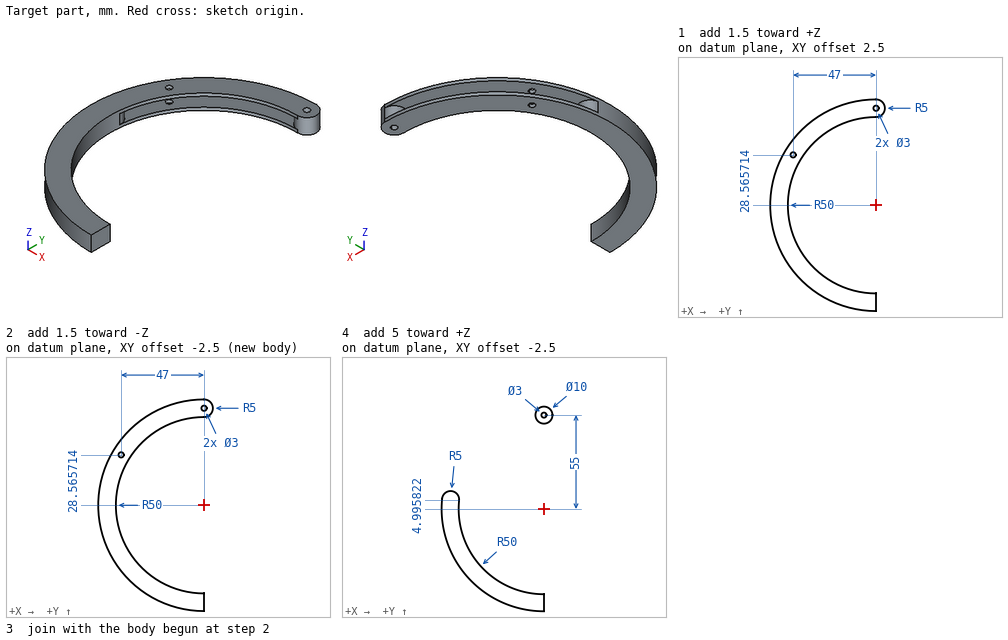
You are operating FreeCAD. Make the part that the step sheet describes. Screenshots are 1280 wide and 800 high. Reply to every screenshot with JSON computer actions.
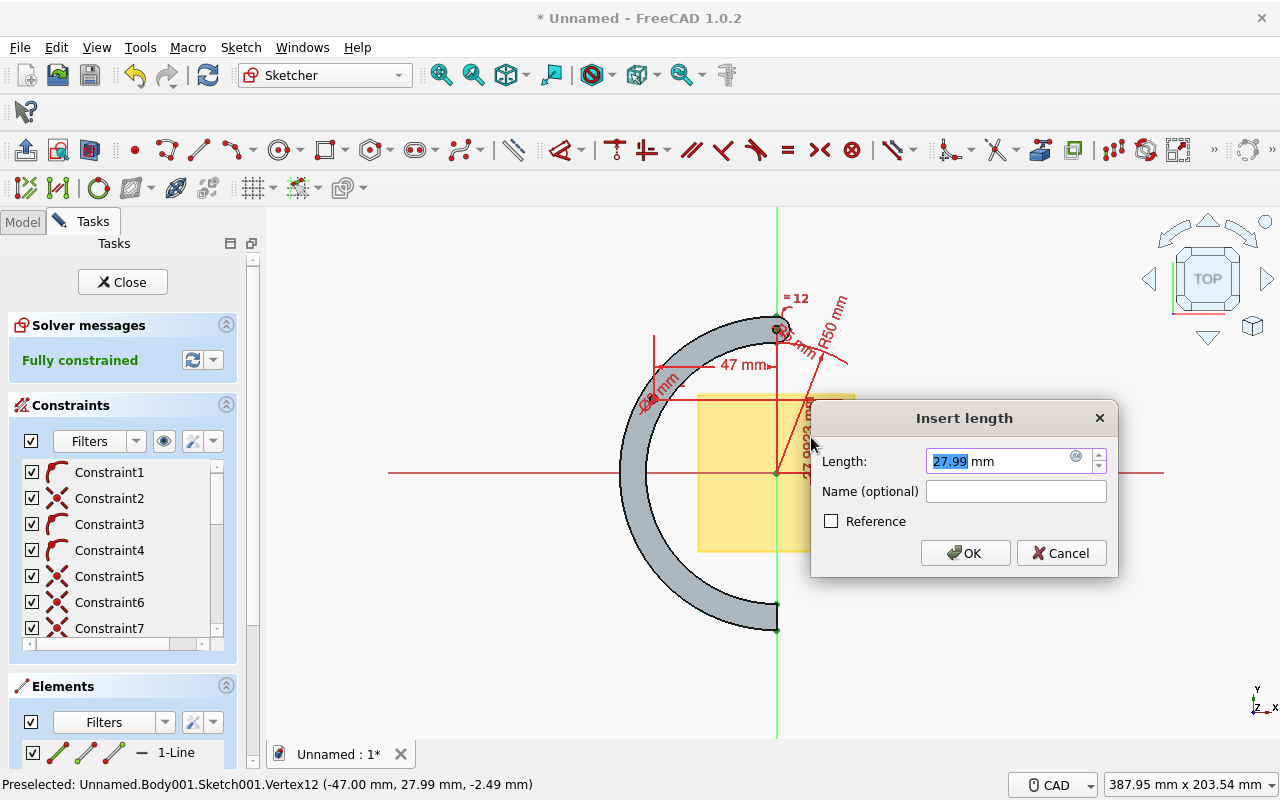
{"action": "type", "text": "28.565714"}
{"action": "key", "text": "Return"}
{"action": "key", "text": "Escape"}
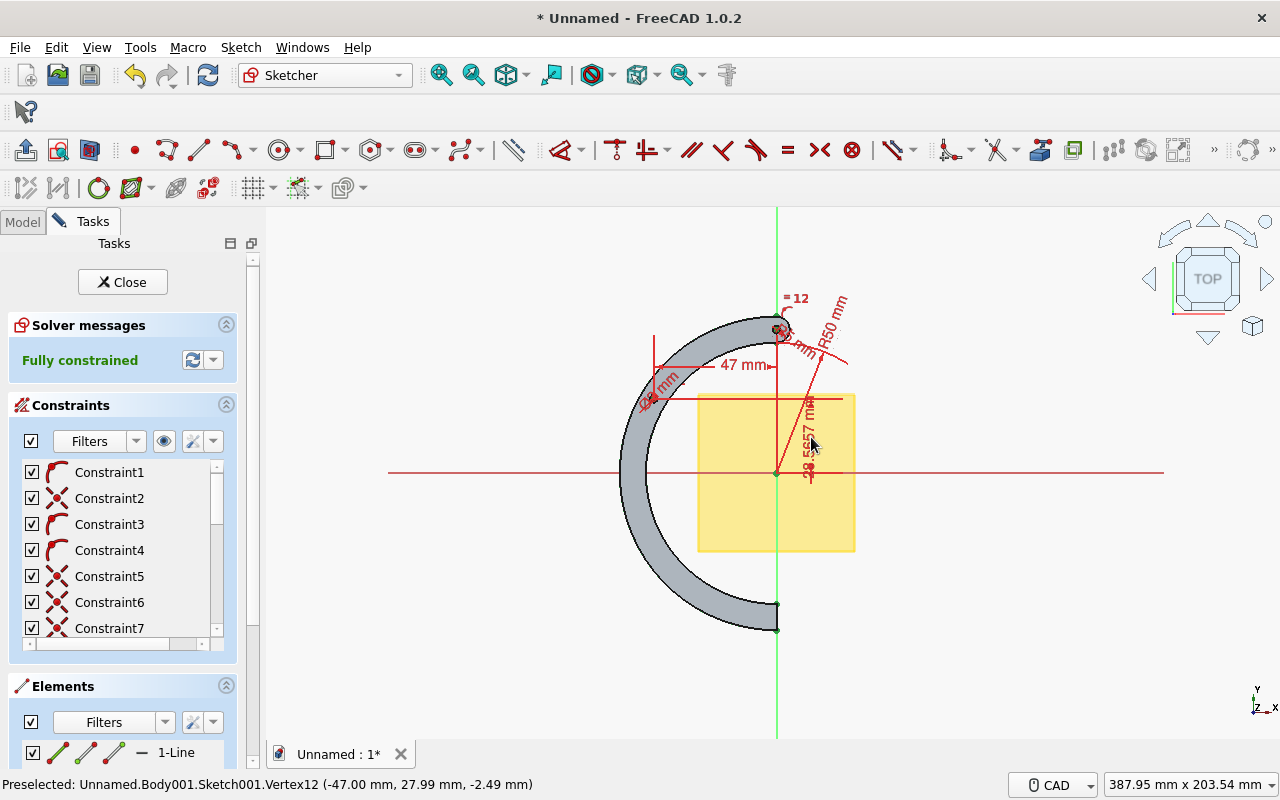
{"action": "left_click", "coordinate": [123, 282]}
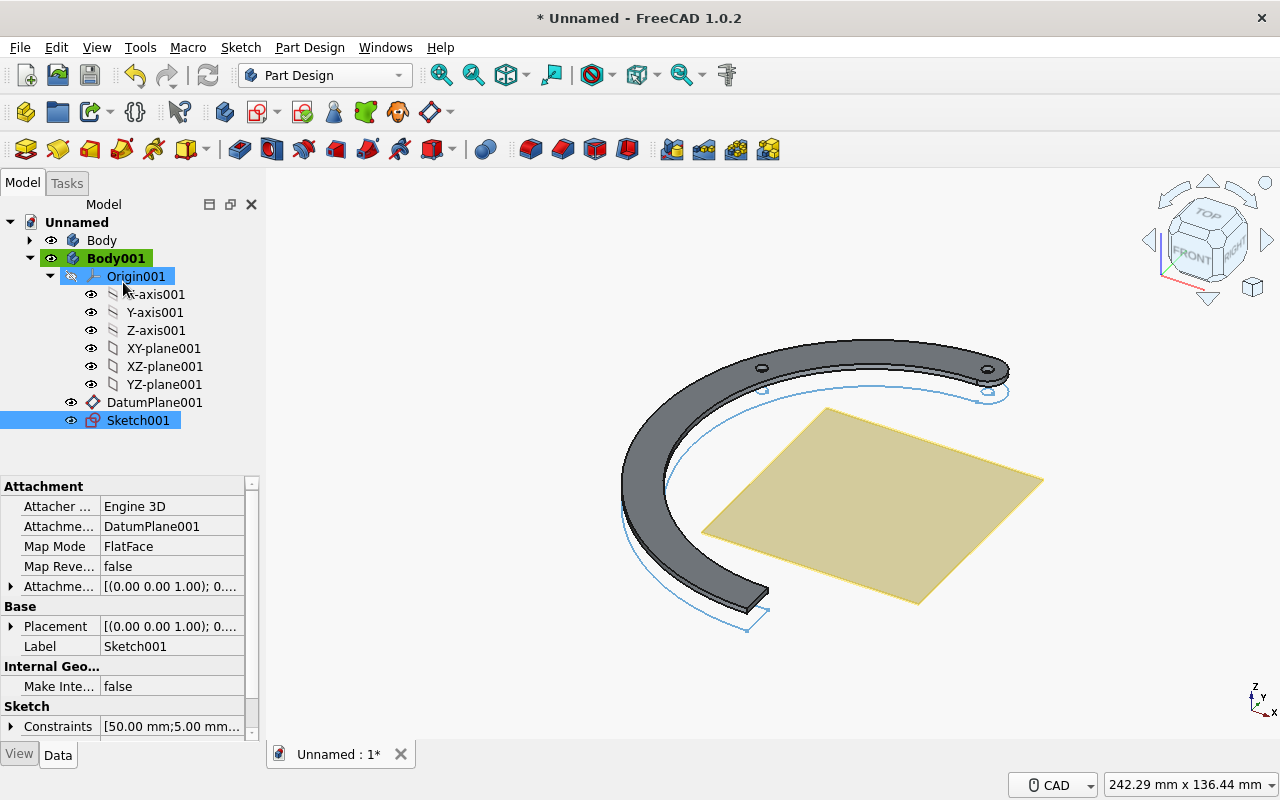
{"action": "left_click", "coordinate": [26, 150]}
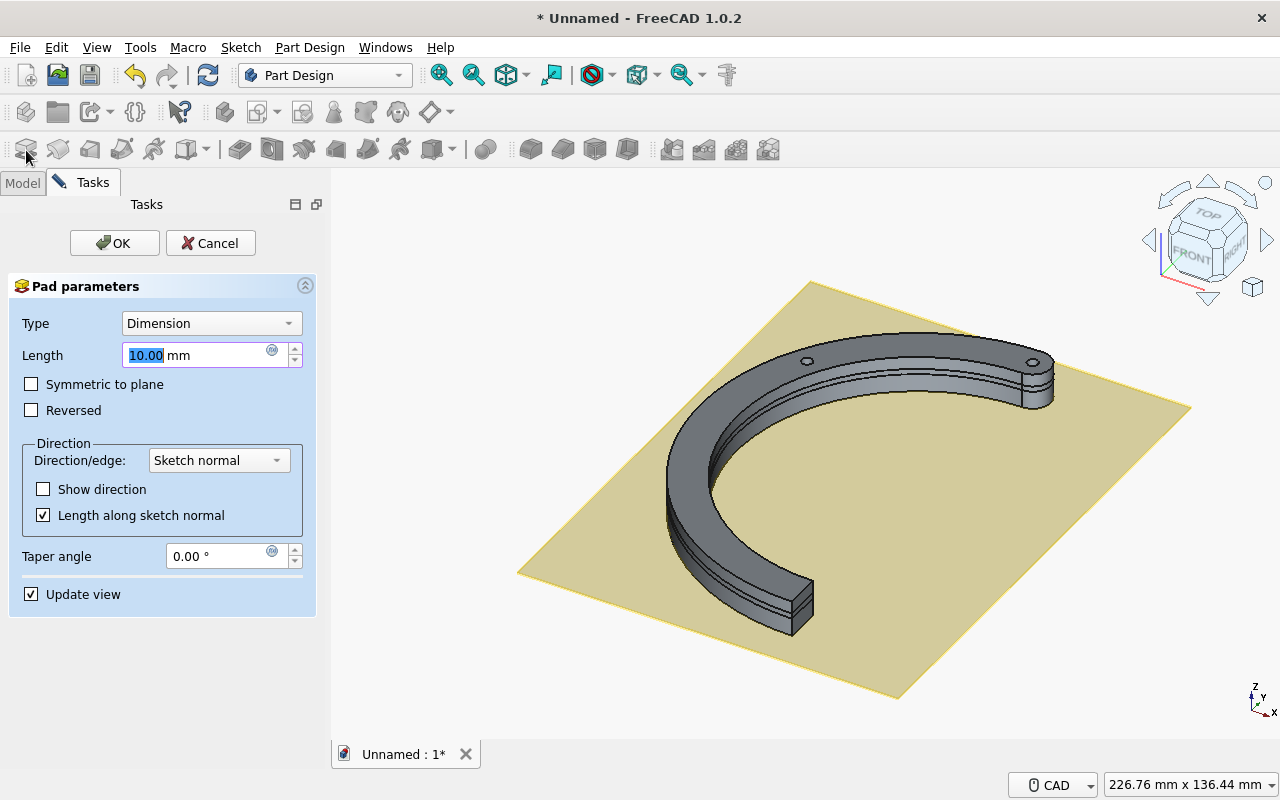
{"action": "type", "text": "1.5"}
{"action": "key", "text": "Tab"}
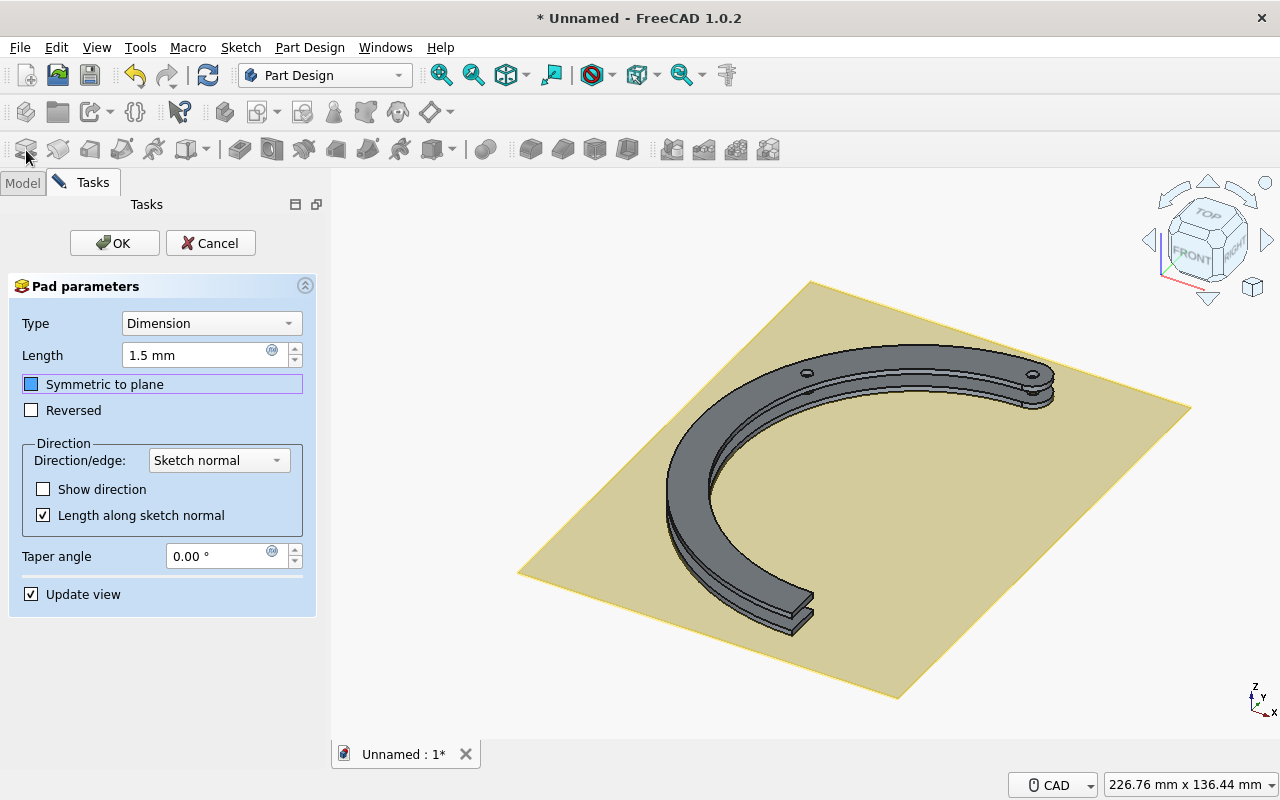
{"action": "left_click", "coordinate": [30, 410]}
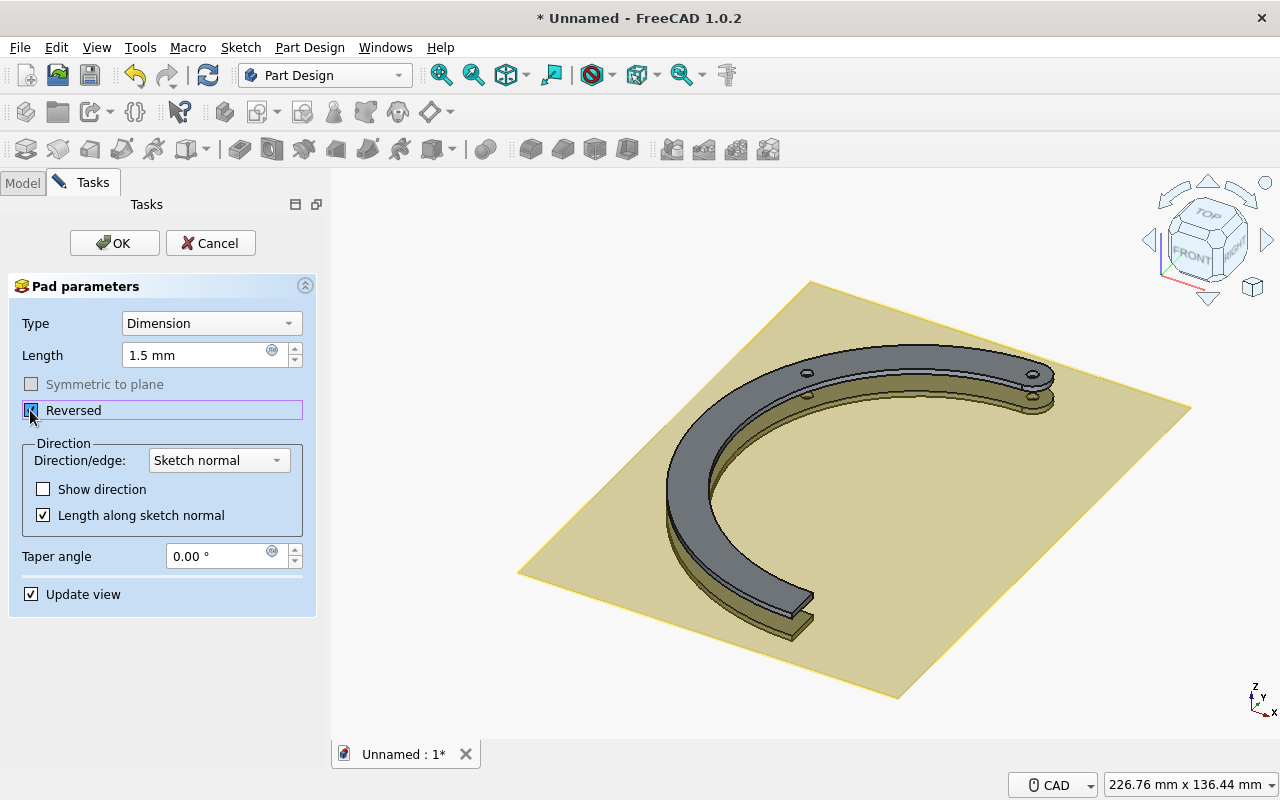
{"action": "left_click", "coordinate": [115, 243]}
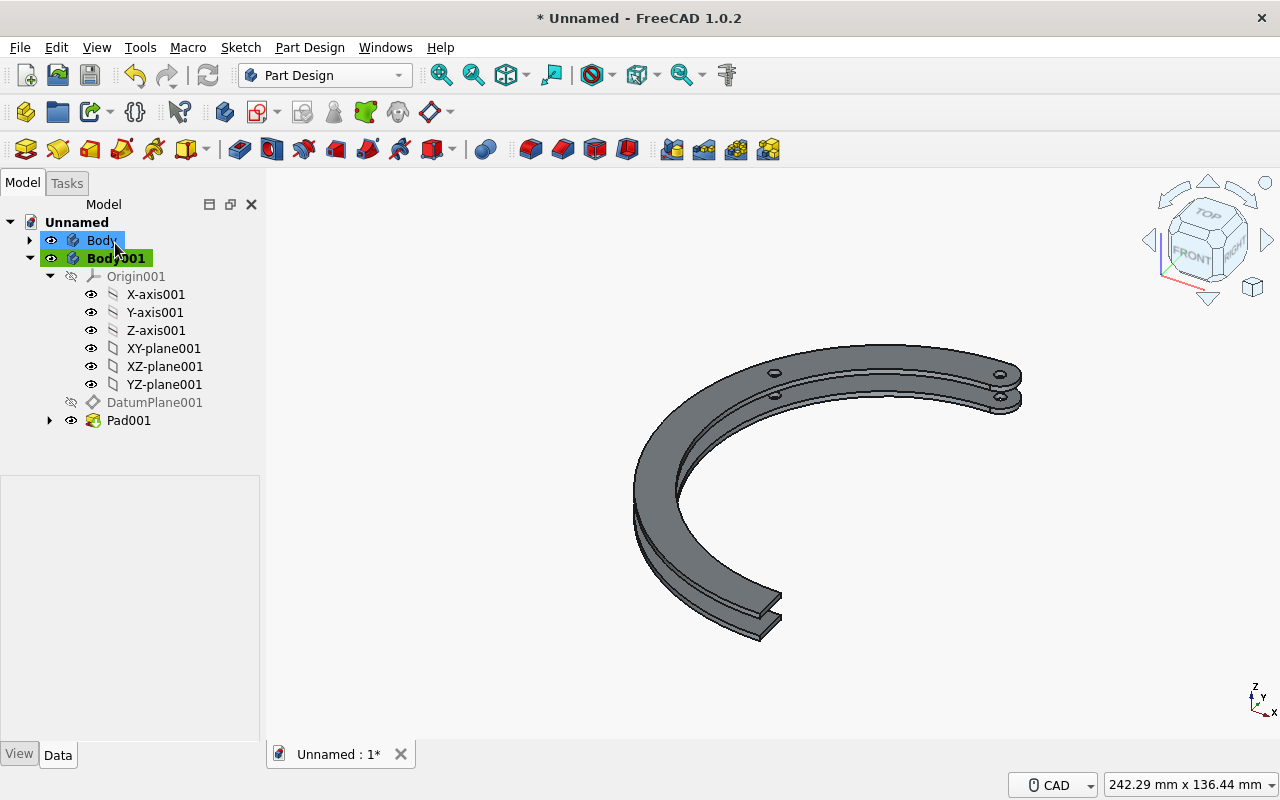
{"action": "double_click", "coordinate": [96, 240]}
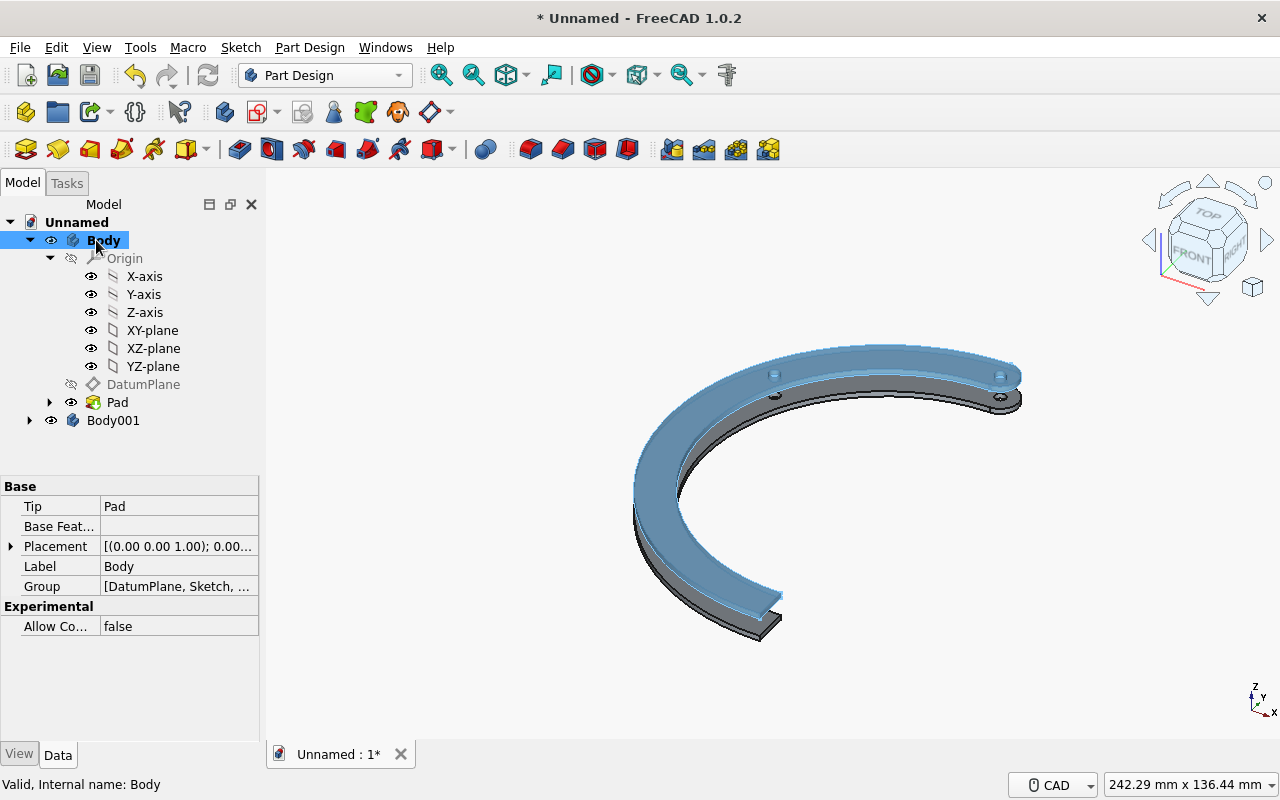
{"action": "left_click", "coordinate": [96, 240]}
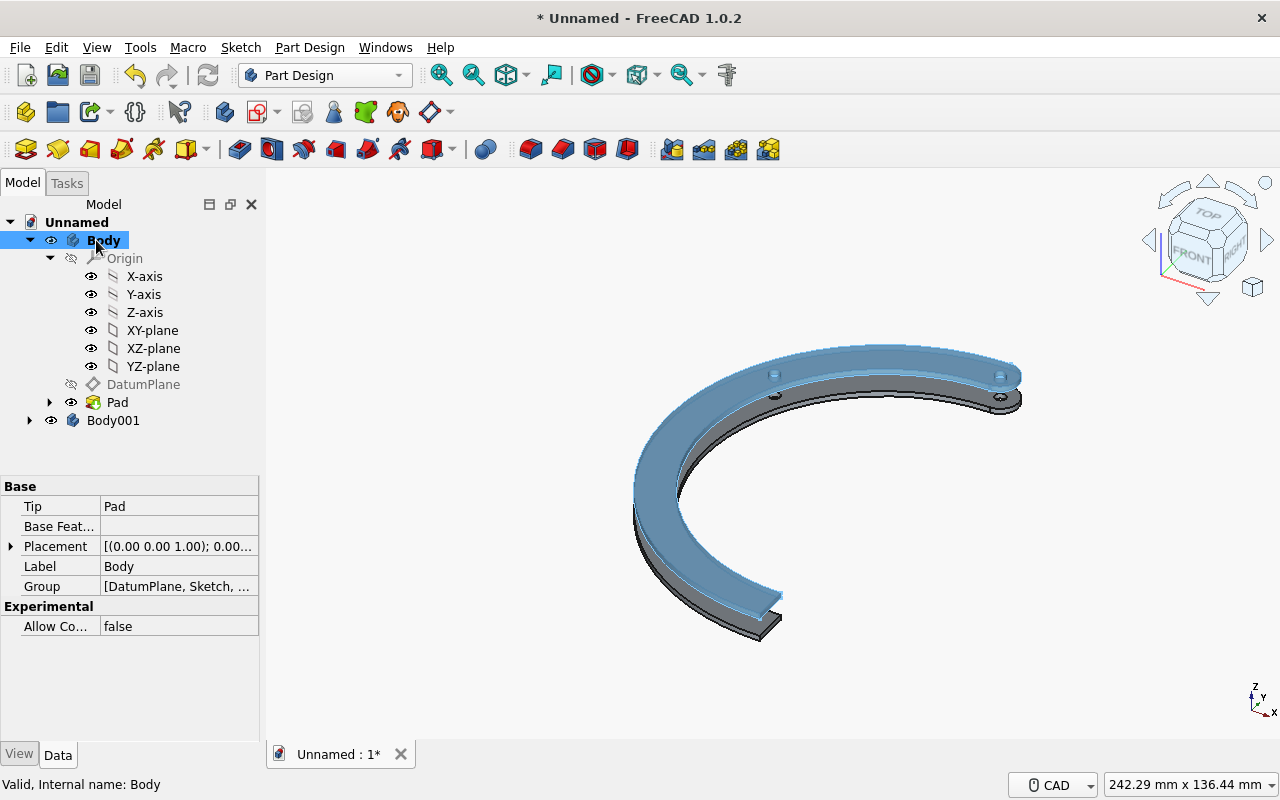
{"action": "left_click", "coordinate": [146, 626]}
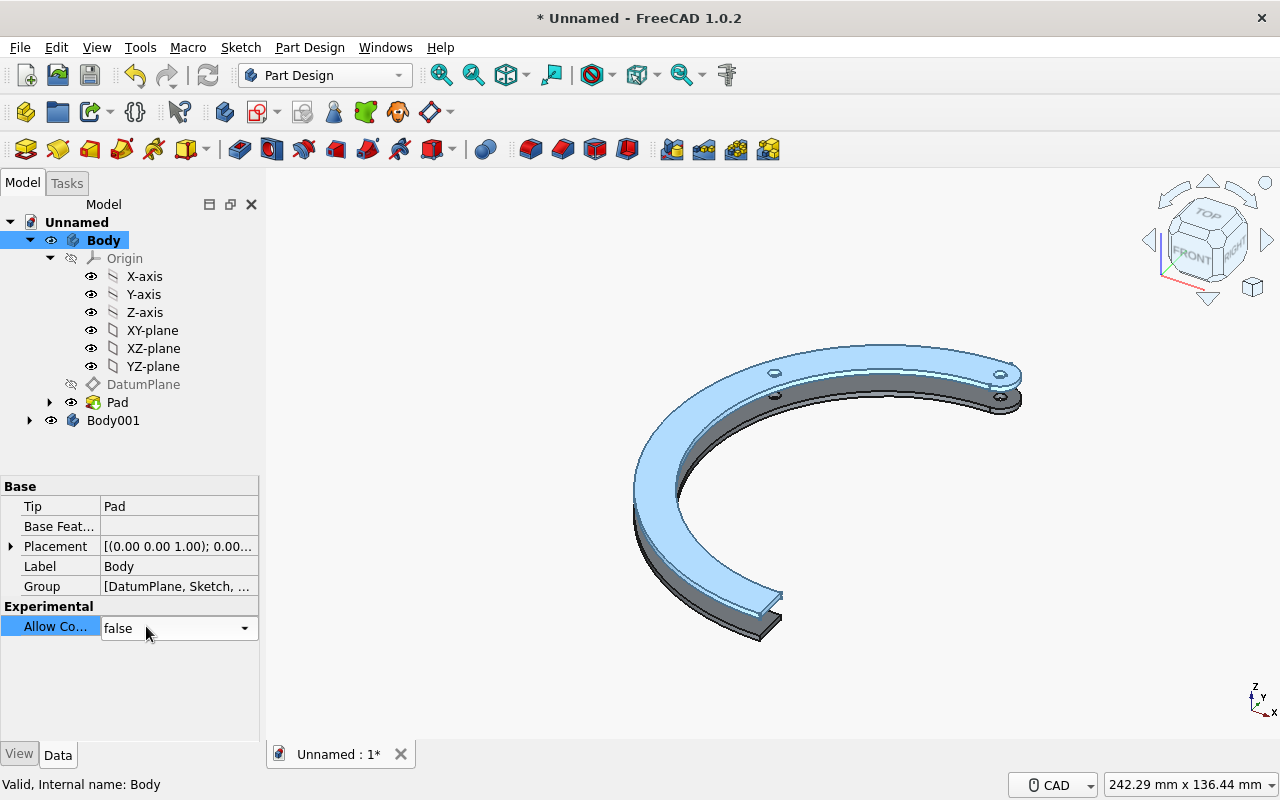
{"action": "left_click", "coordinate": [146, 626]}